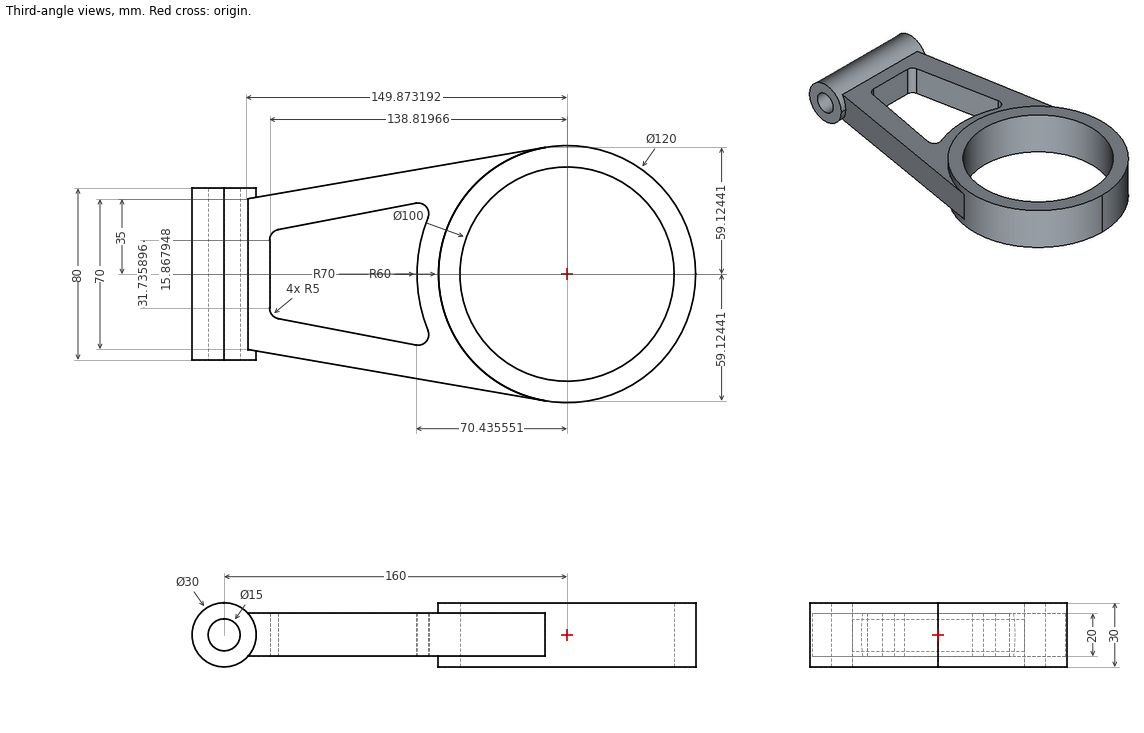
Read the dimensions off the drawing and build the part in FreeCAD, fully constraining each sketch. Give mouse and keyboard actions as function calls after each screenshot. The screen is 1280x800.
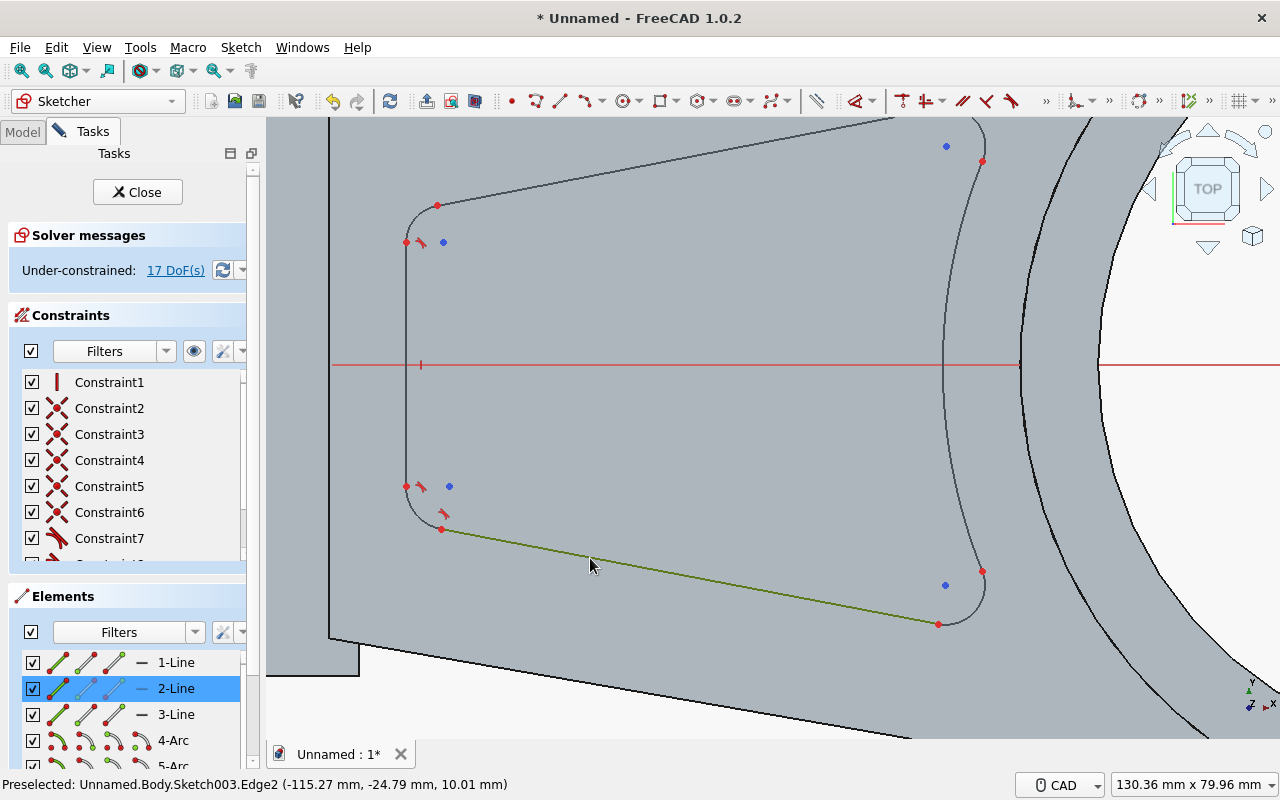
click(963, 621)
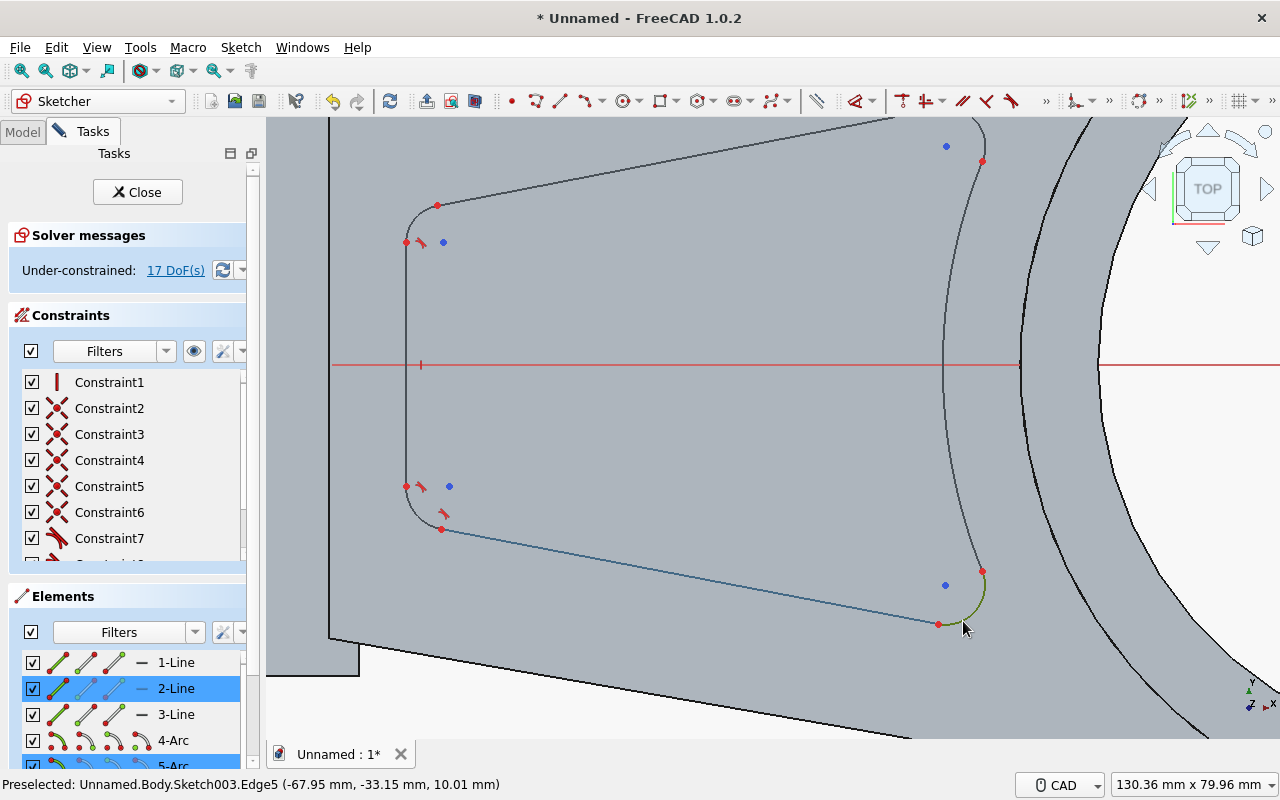
click(1012, 102)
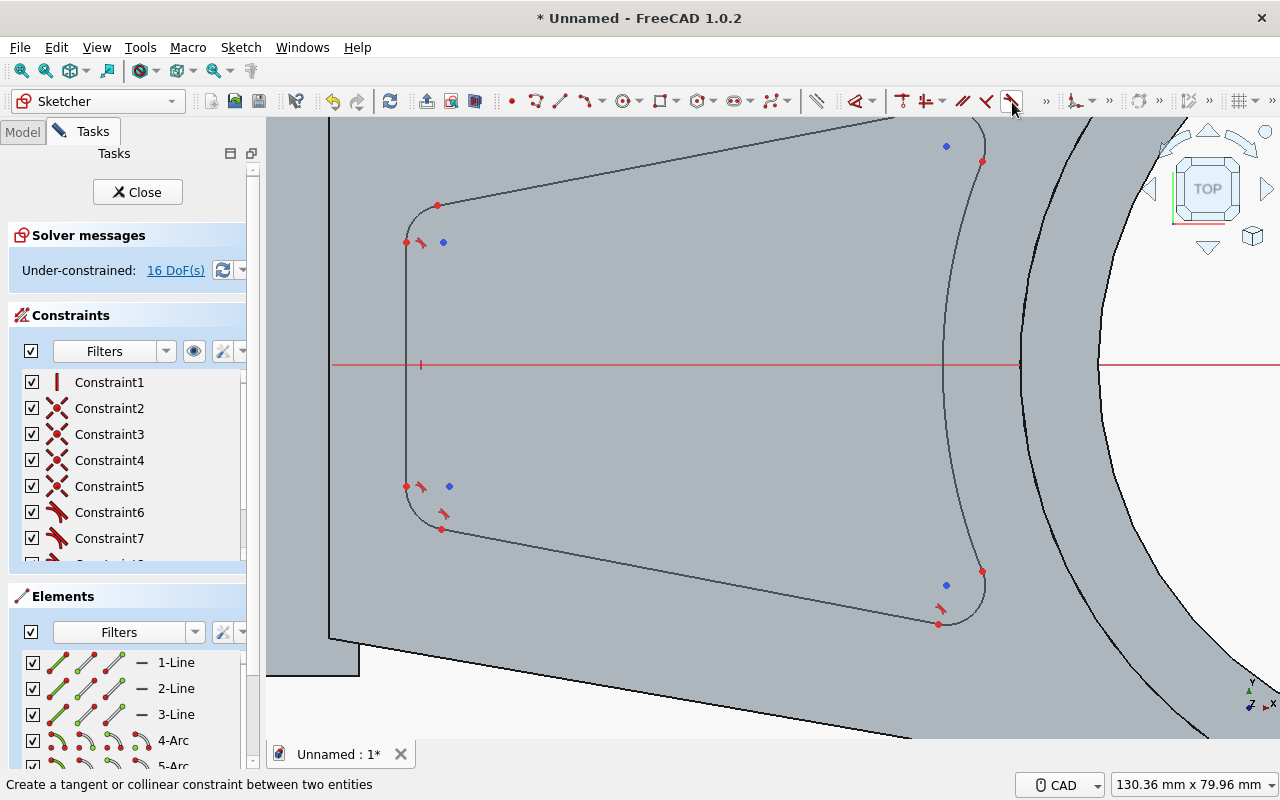
click(588, 177)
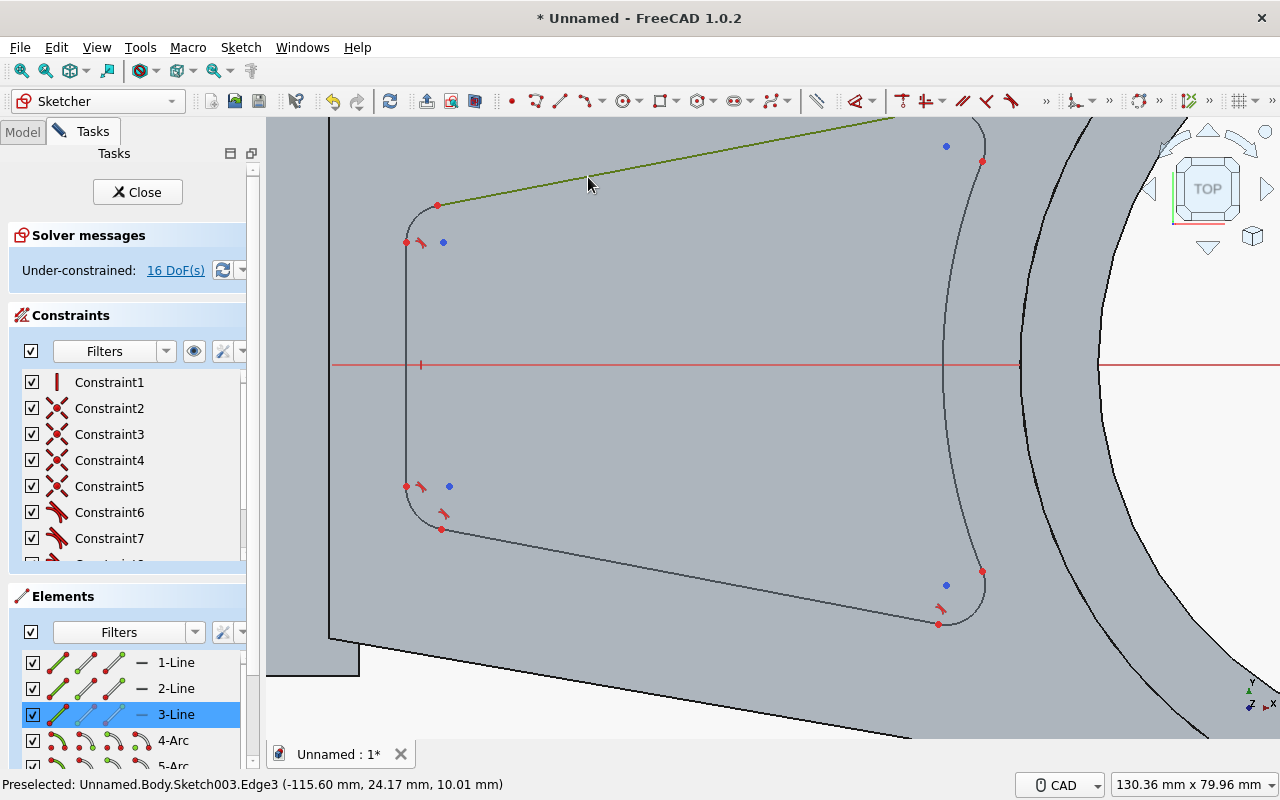
click(985, 145)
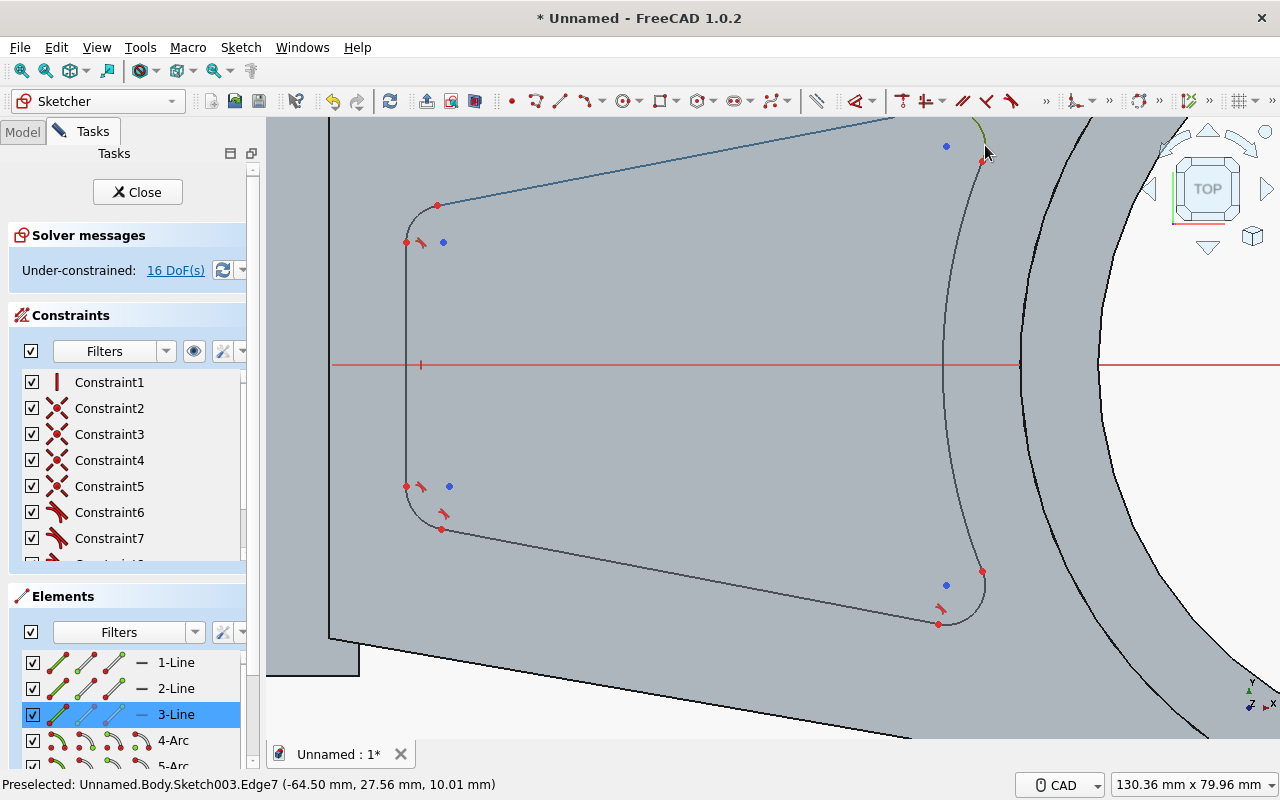
click(1012, 102)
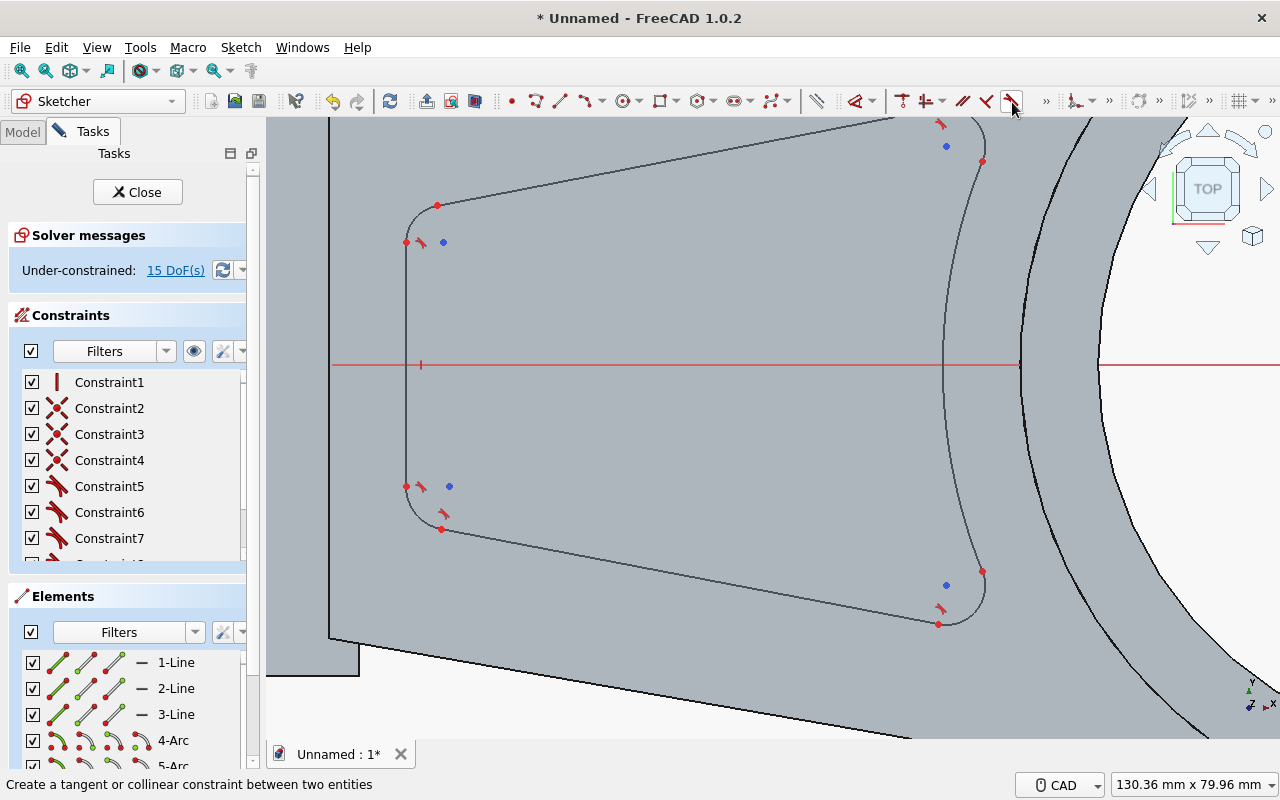
click(588, 177)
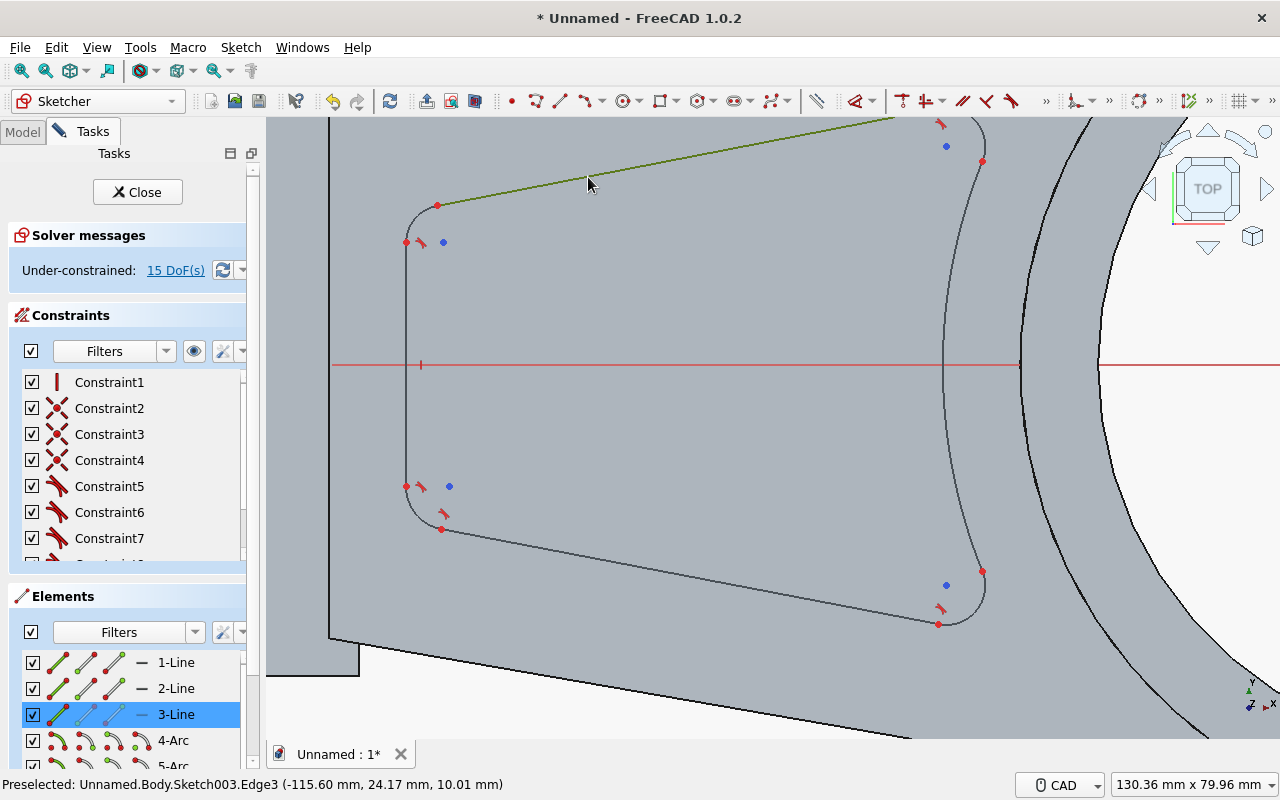
click(423, 212)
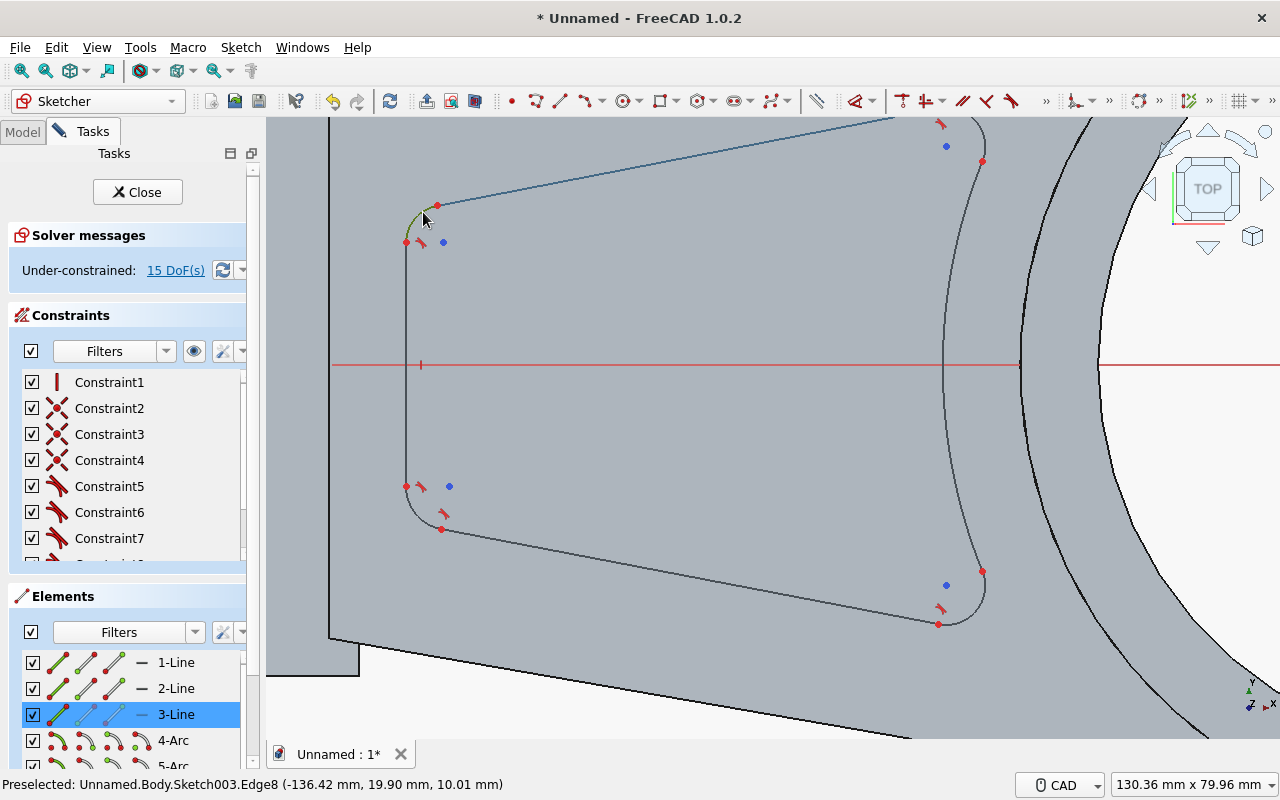
click(1012, 102)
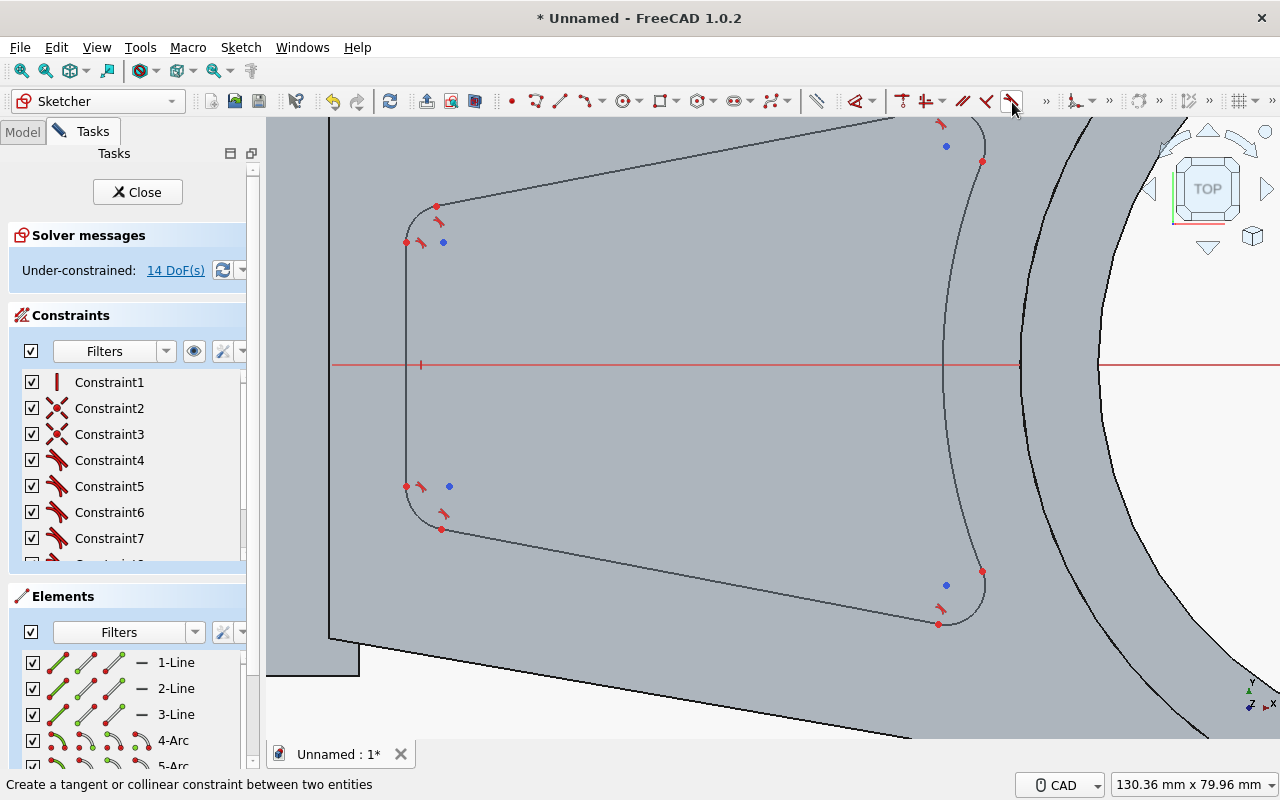
click(963, 621)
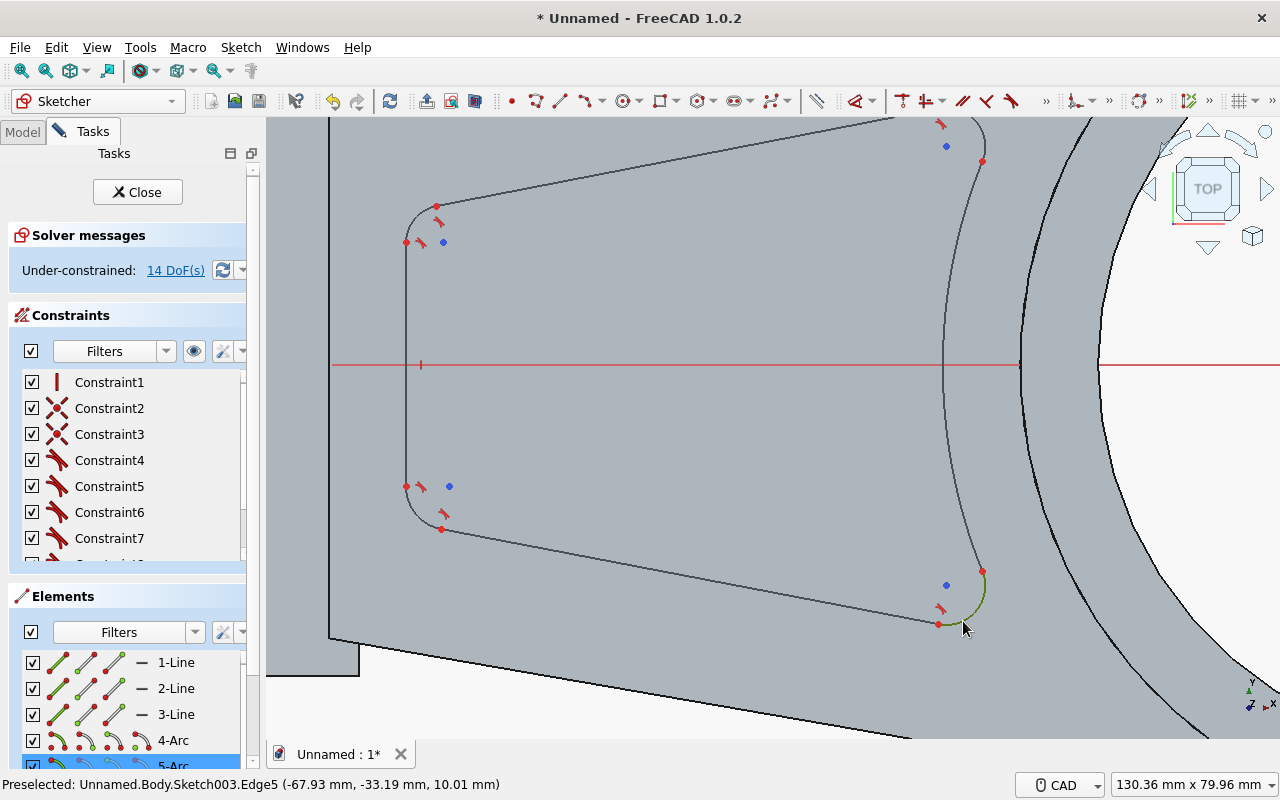
click(949, 283)